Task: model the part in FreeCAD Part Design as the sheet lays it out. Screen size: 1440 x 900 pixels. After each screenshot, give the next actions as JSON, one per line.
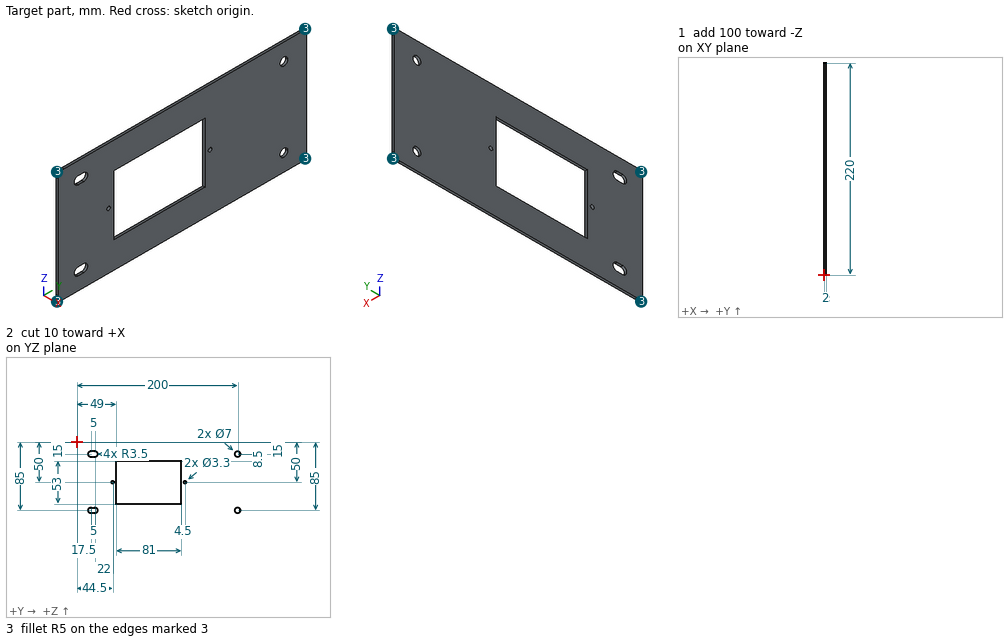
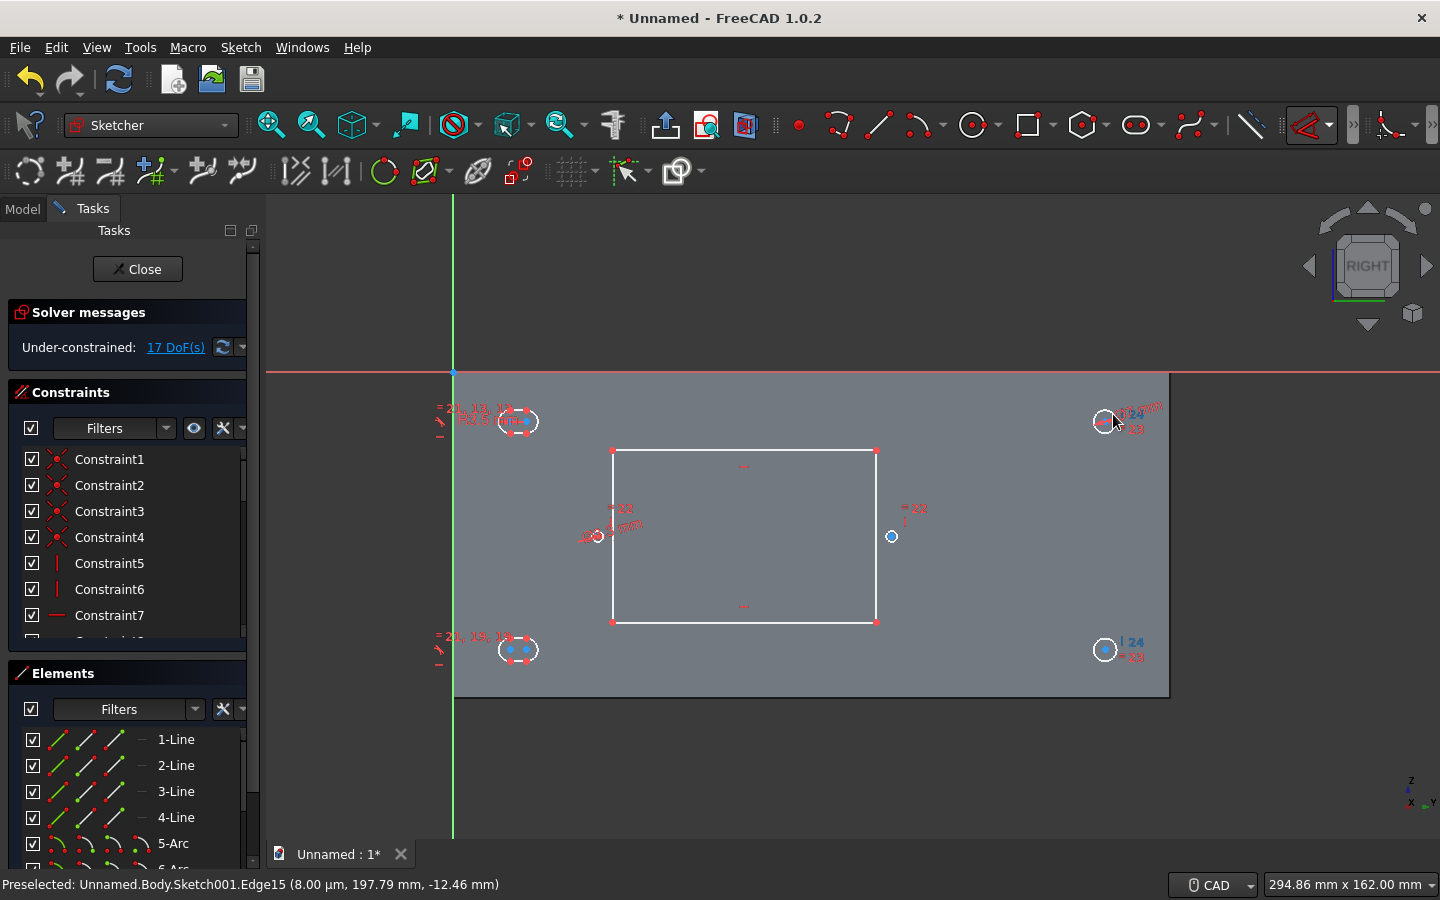
{"action": "scroll", "coordinate": [517, 410], "scroll_direction": "up", "scroll_amount": 5}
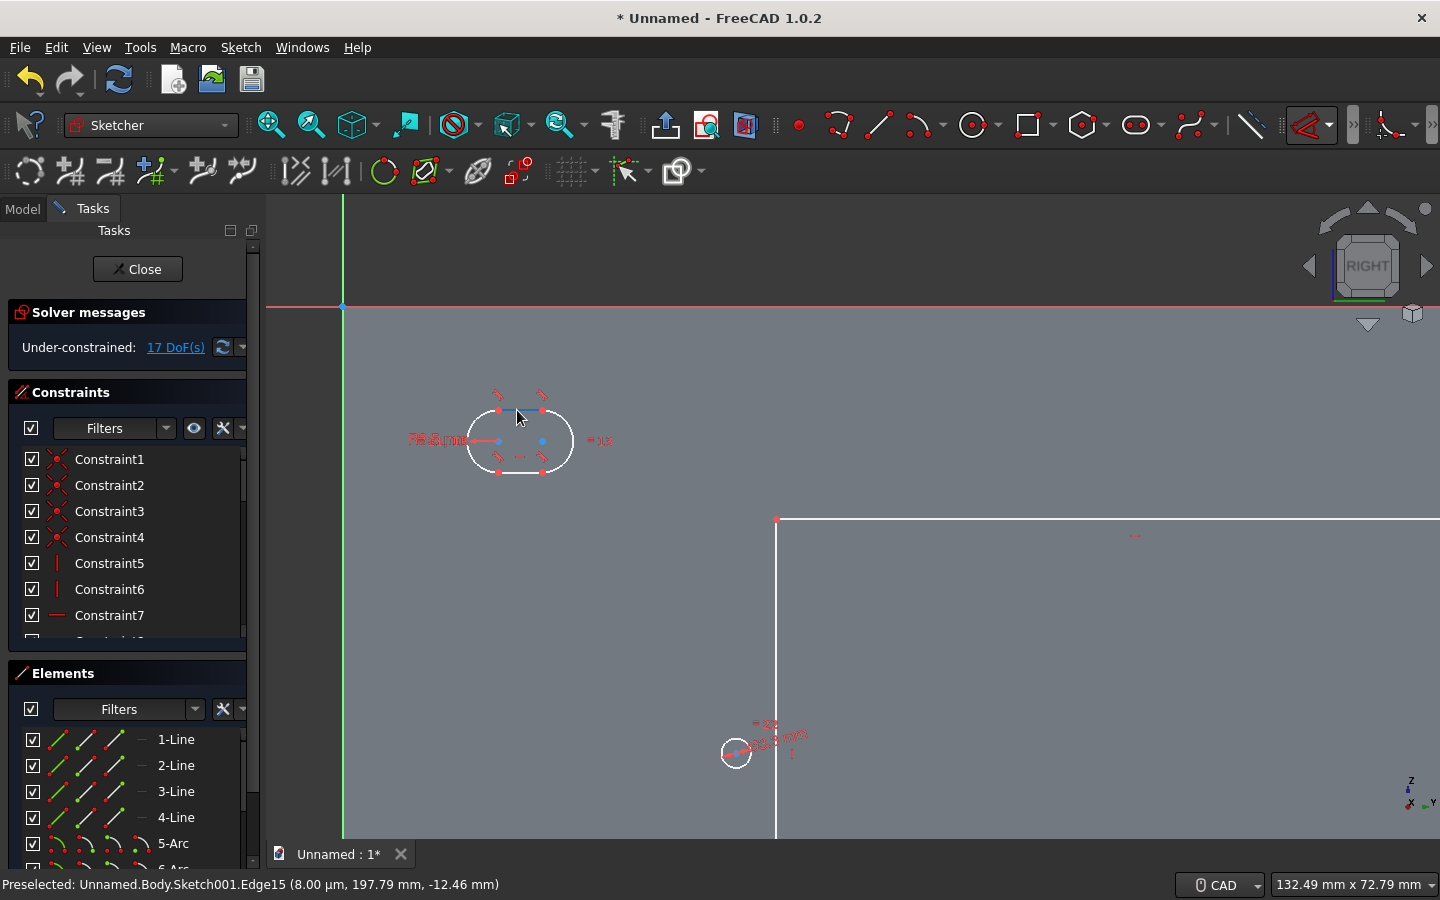
{"action": "left_click", "coordinate": [516, 410]}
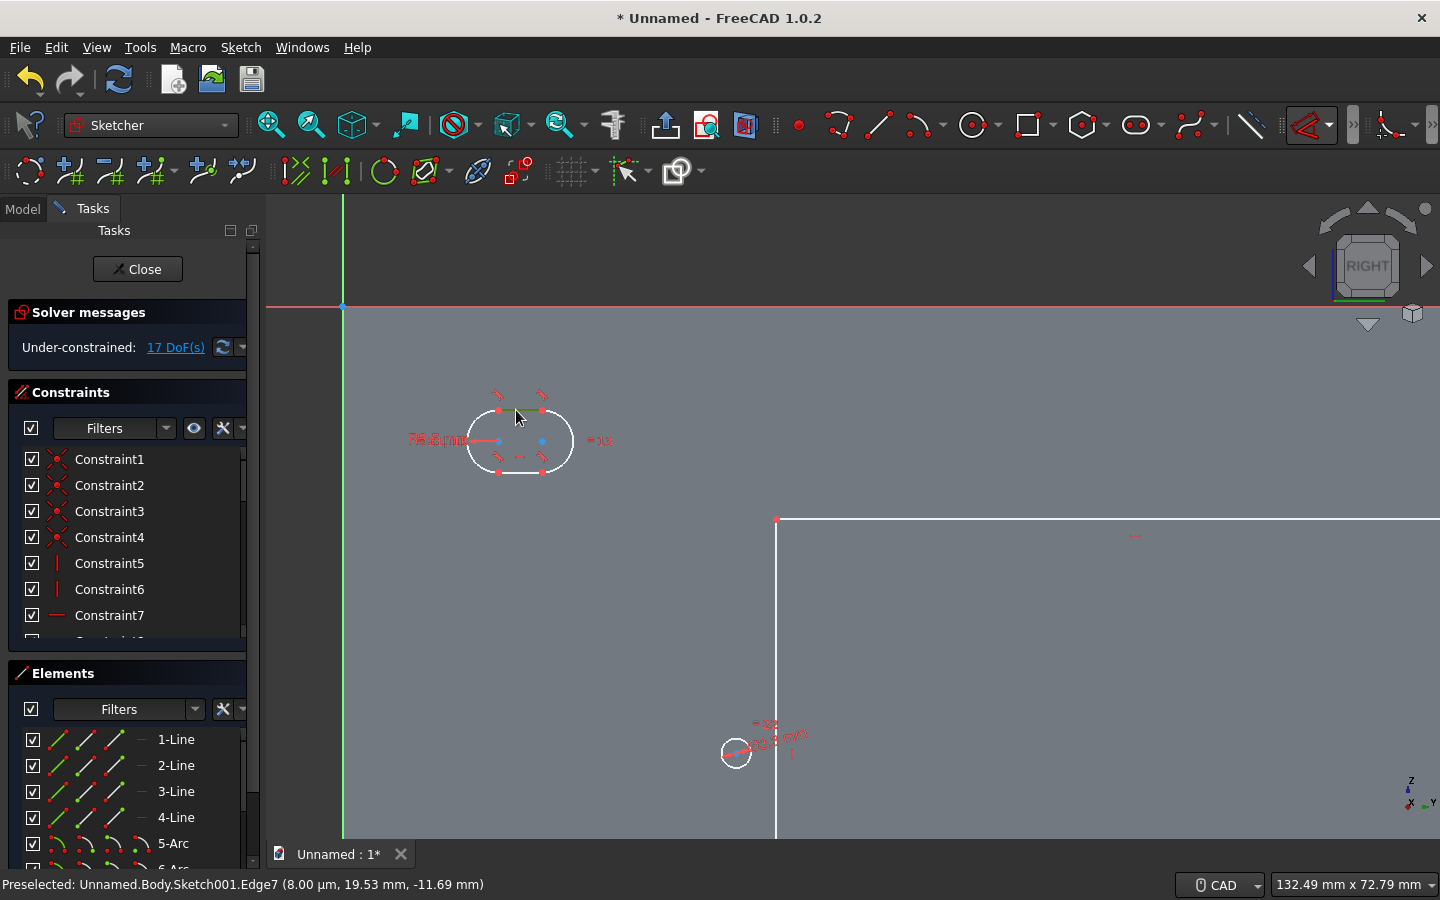
{"action": "left_click", "coordinate": [1332, 126]}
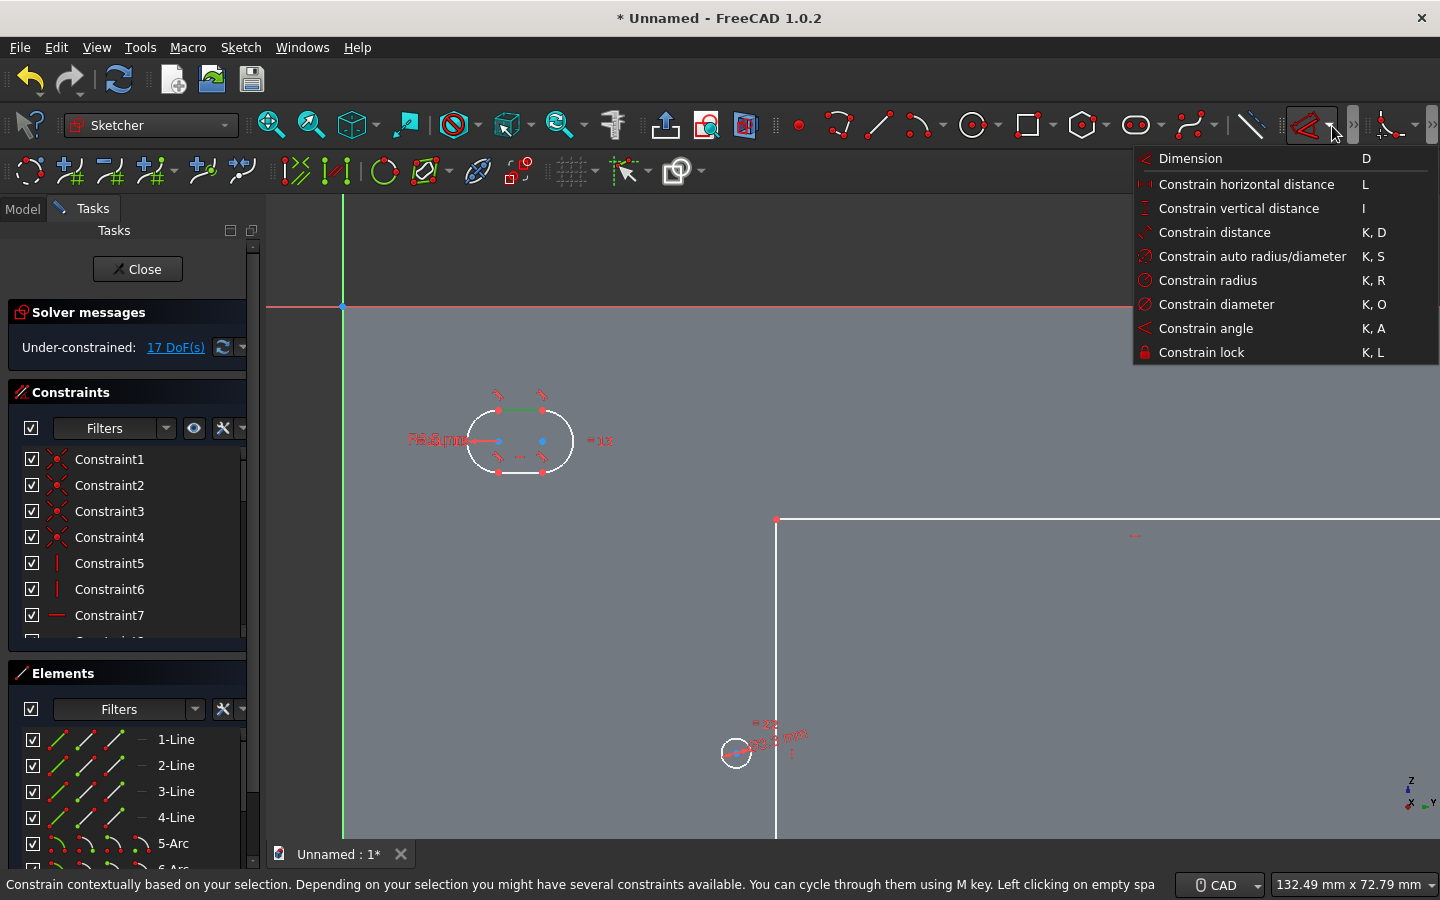
{"action": "left_click", "coordinate": [1286, 184]}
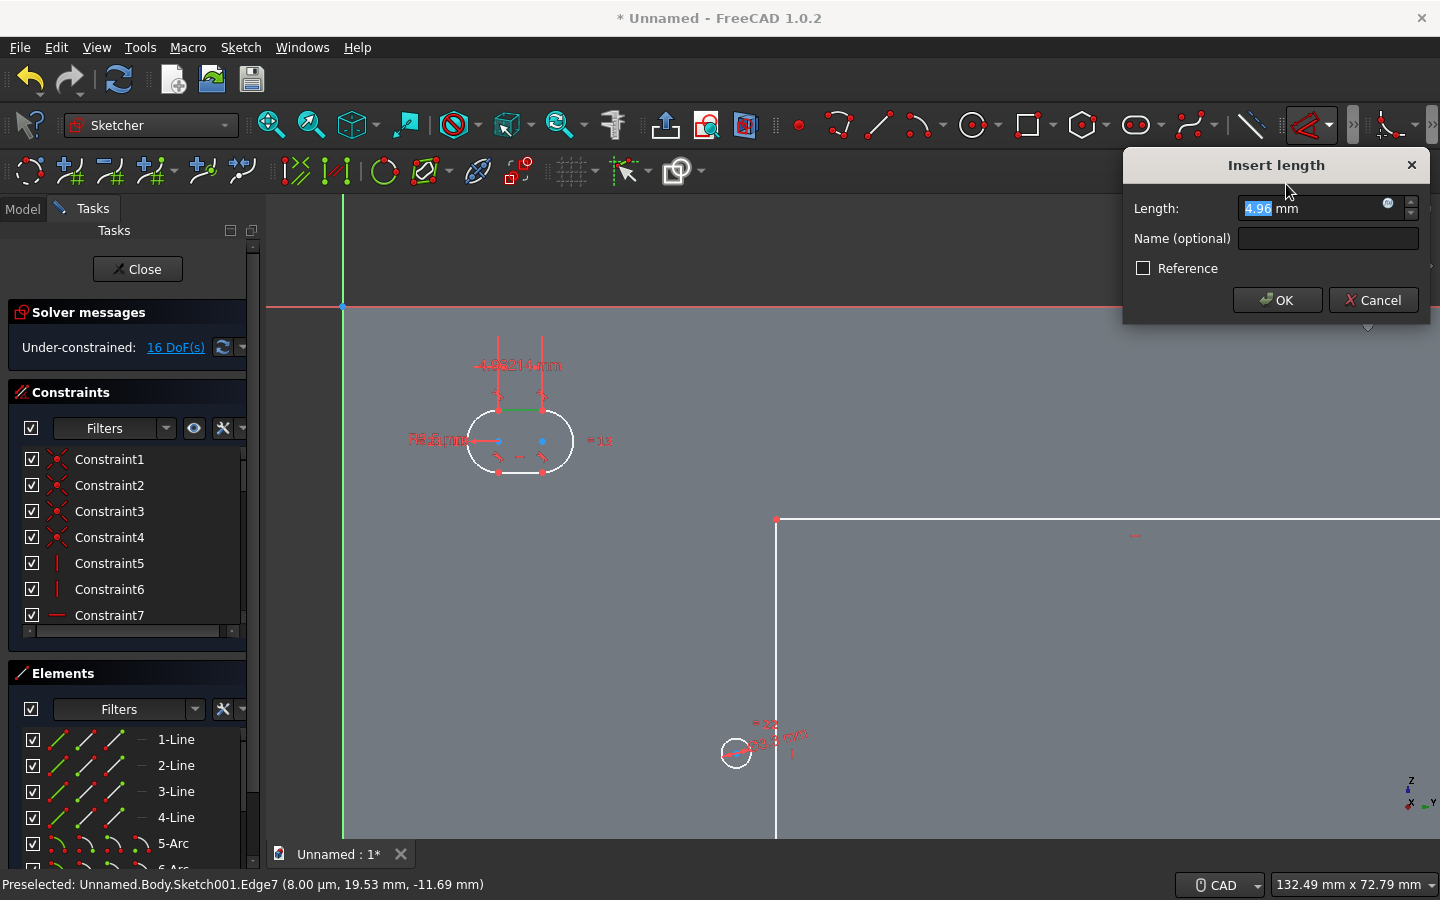
{"action": "type", "text": "5"}
{"action": "key", "text": "Return"}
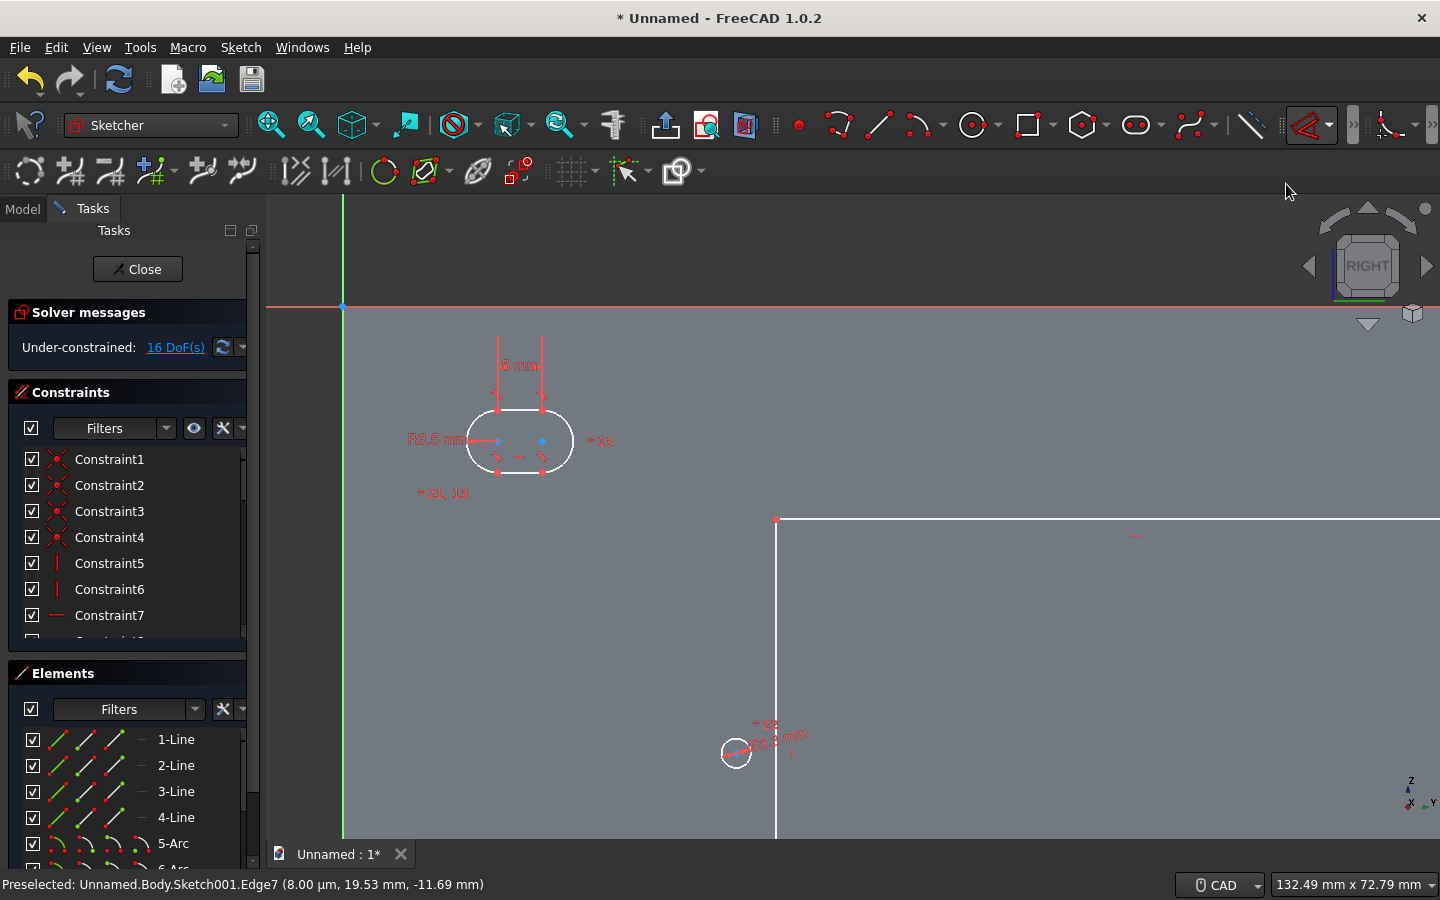
{"action": "scroll", "coordinate": [517, 410], "scroll_direction": "down", "scroll_amount": 5}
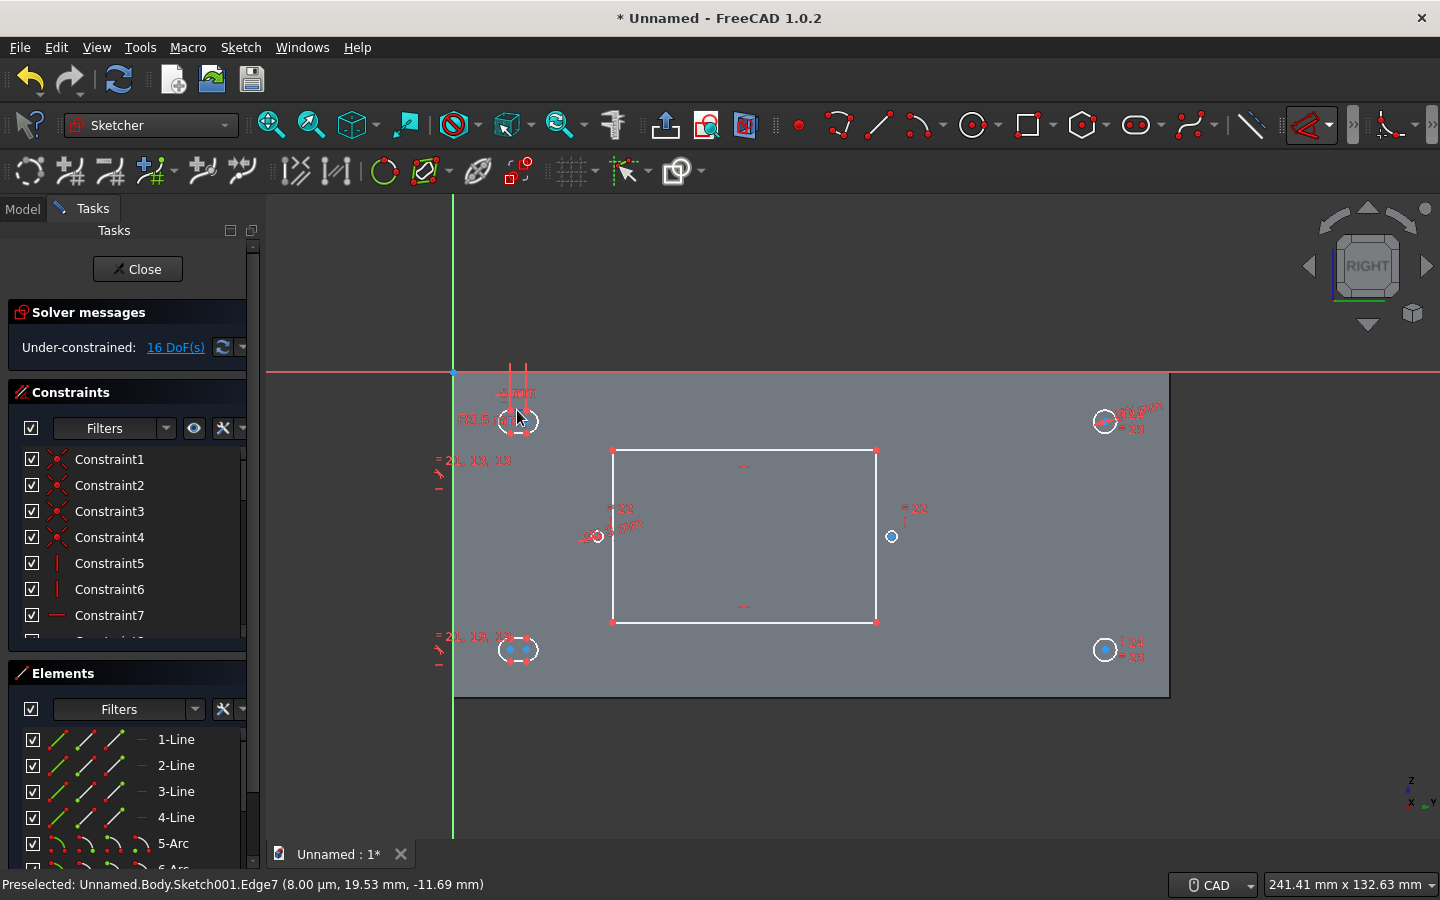
{"action": "scroll", "coordinate": [515, 638], "scroll_direction": "up", "scroll_amount": 6}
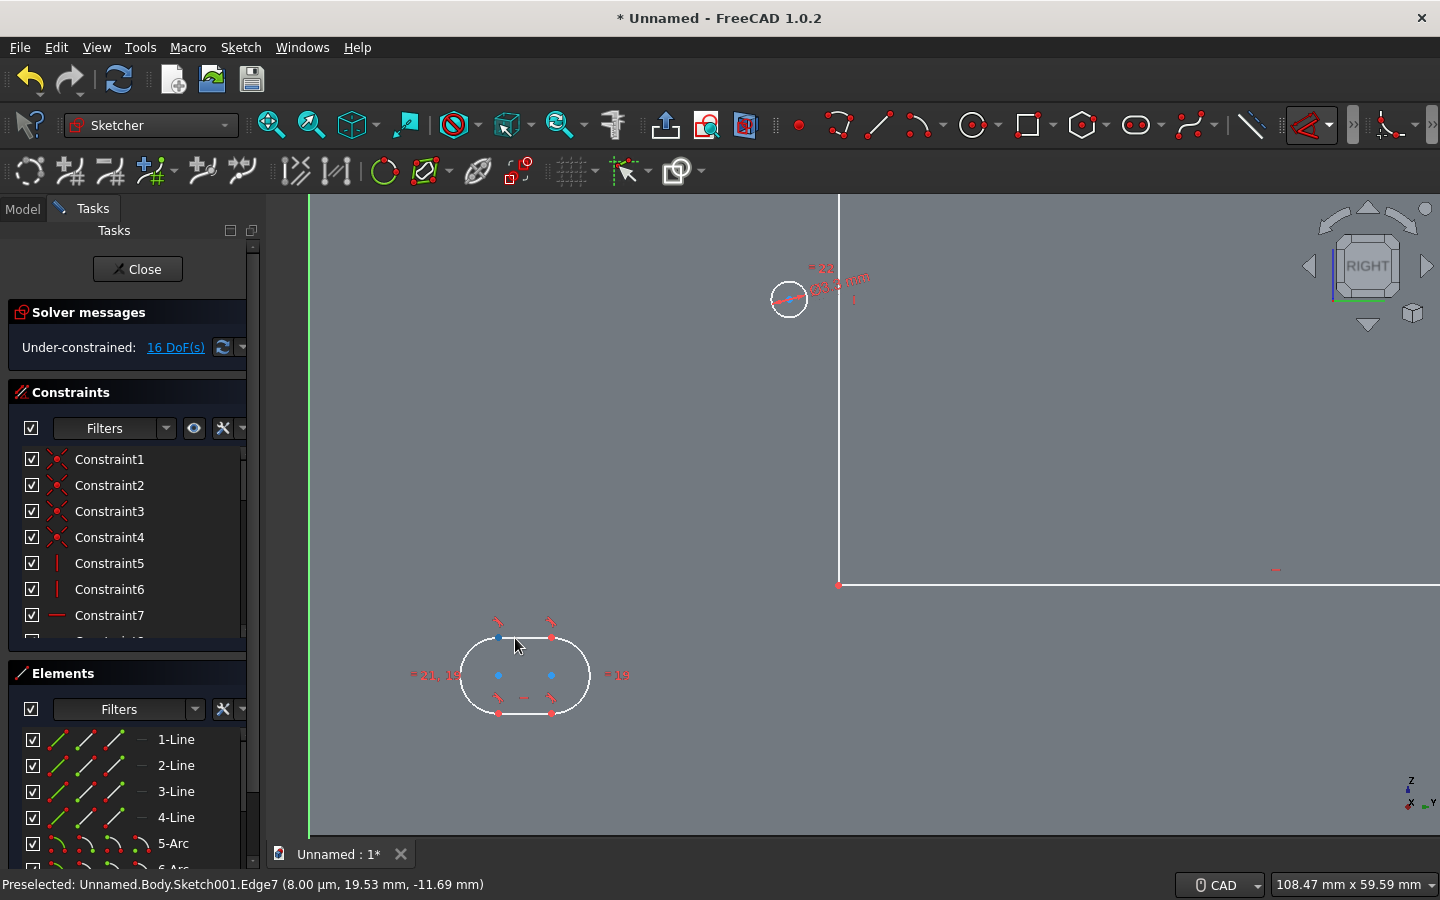
{"action": "left_click", "coordinate": [514, 638]}